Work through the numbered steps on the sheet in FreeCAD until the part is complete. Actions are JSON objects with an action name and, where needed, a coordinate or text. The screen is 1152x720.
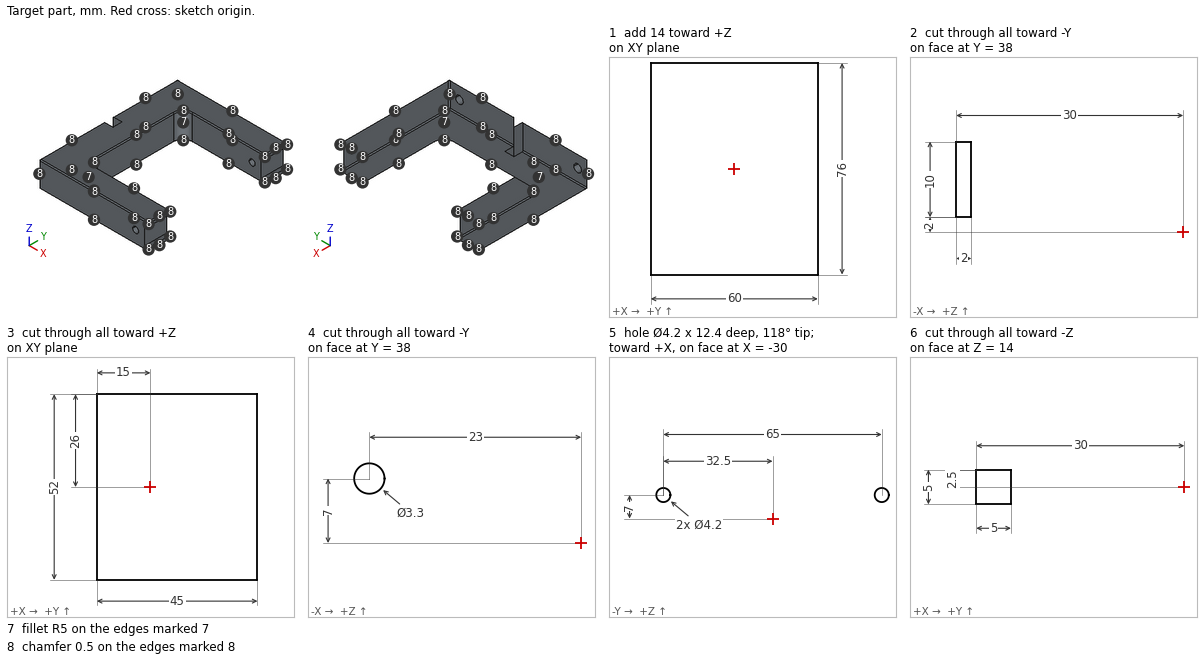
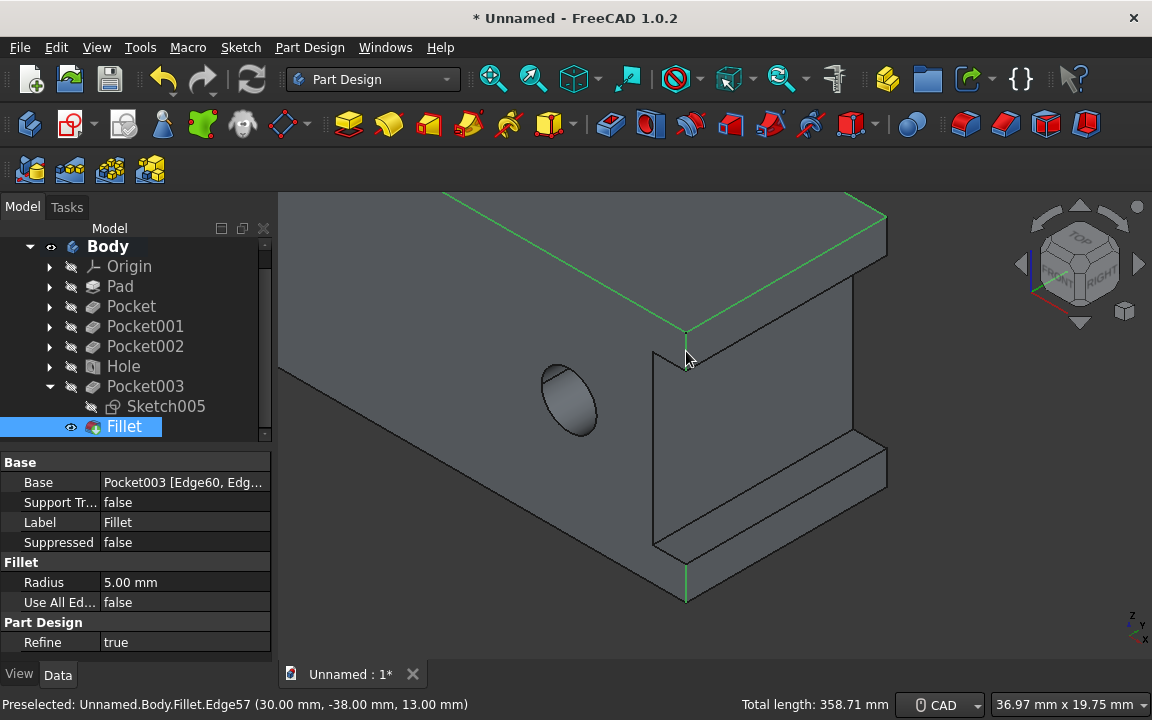
{"action": "key", "text": "v f"}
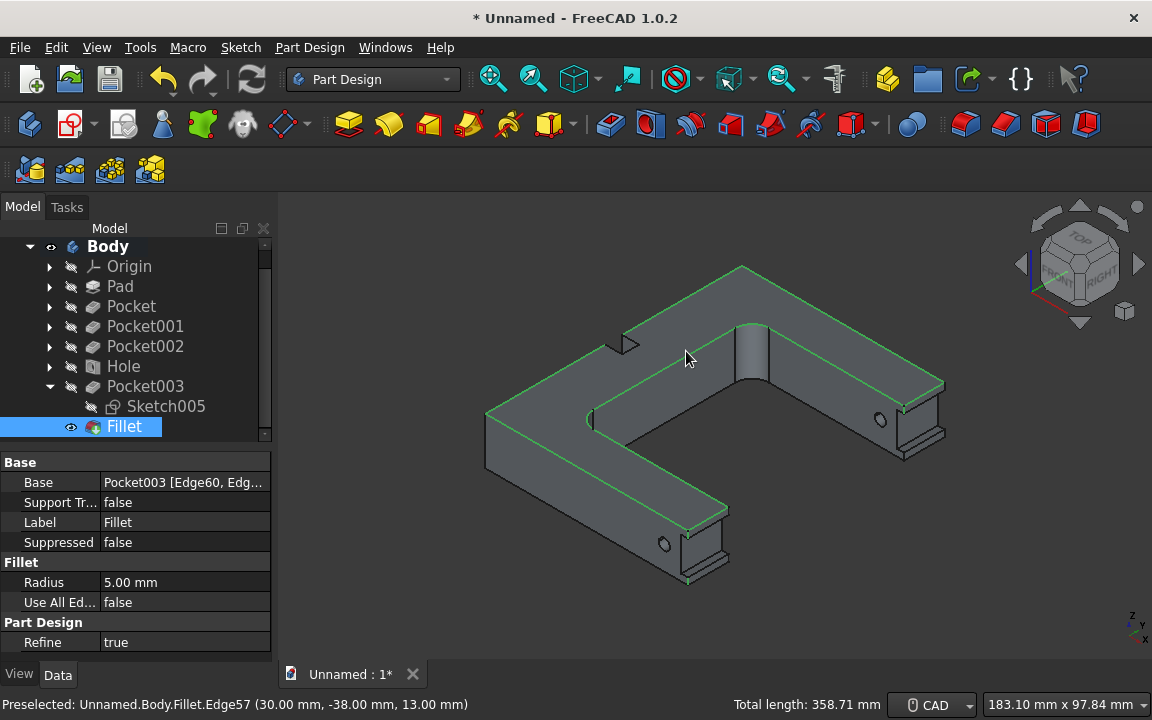
{"action": "key", "text": "1"}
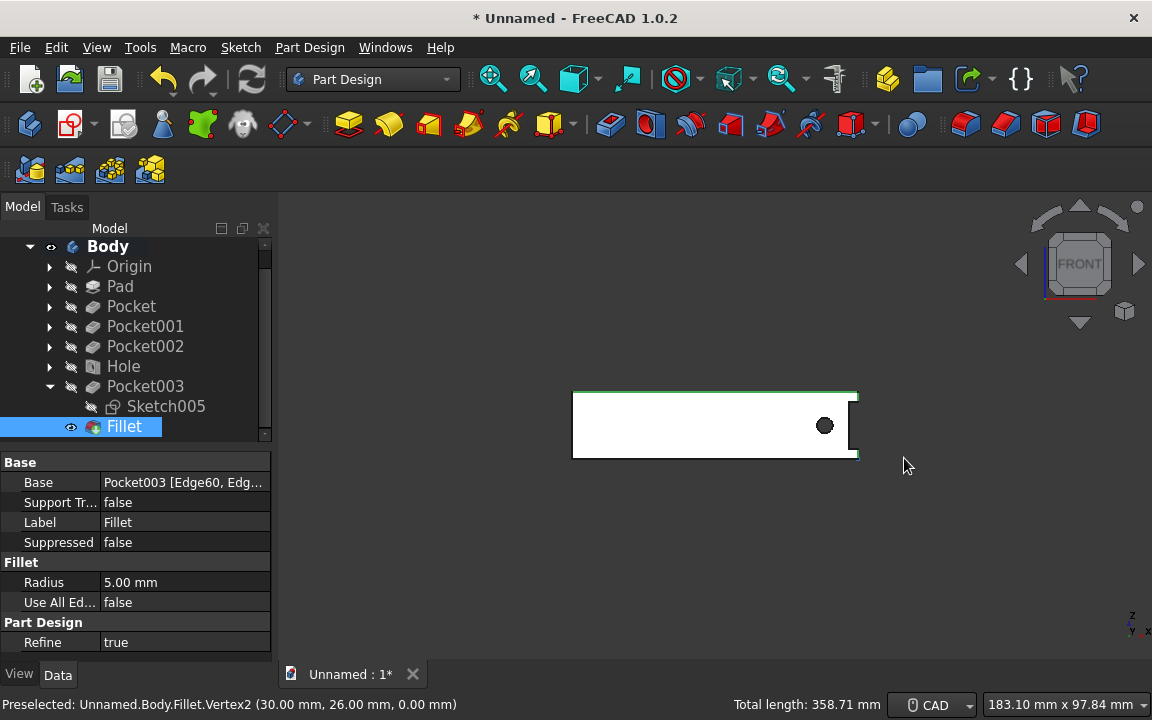
{"action": "key", "text": "v f"}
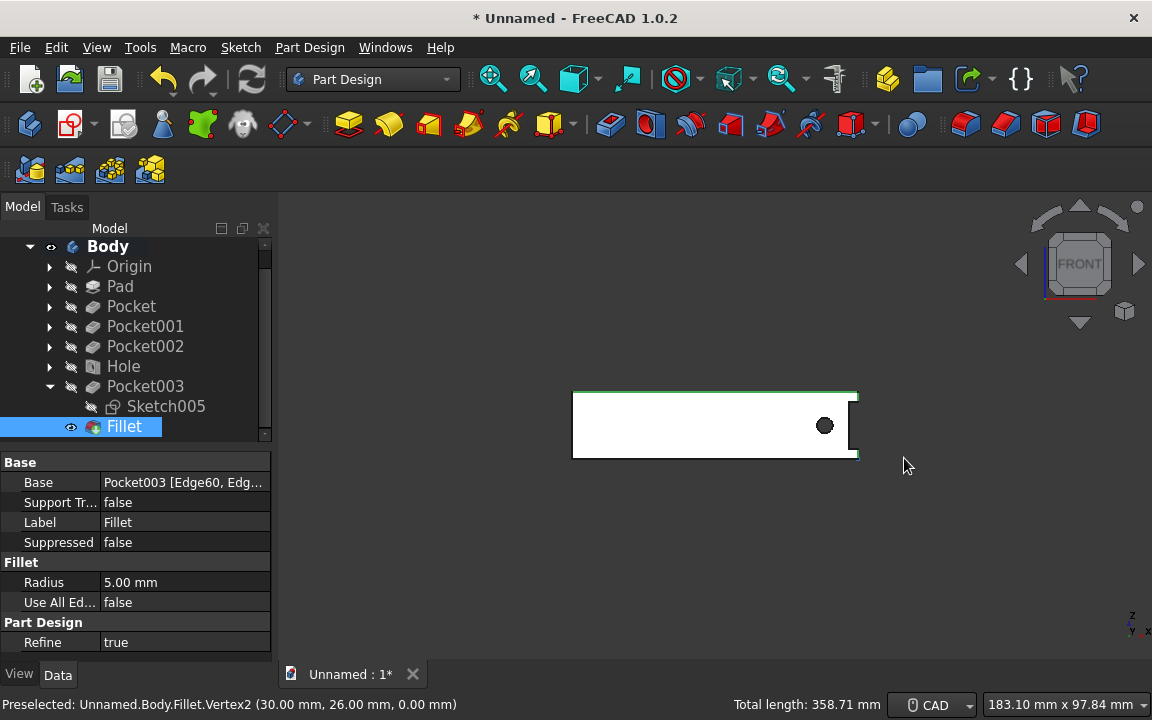
{"action": "left_click", "coordinate": [715, 458], "text": "ctrl"}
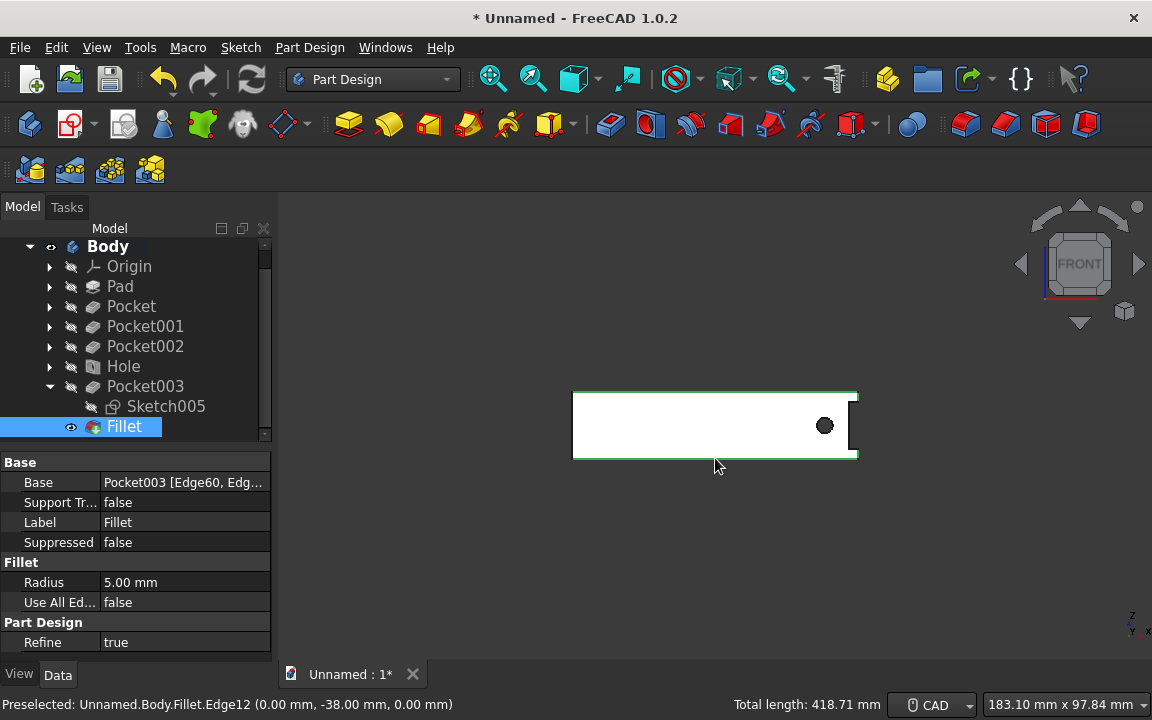
{"action": "left_click", "coordinate": [572, 425], "text": "ctrl"}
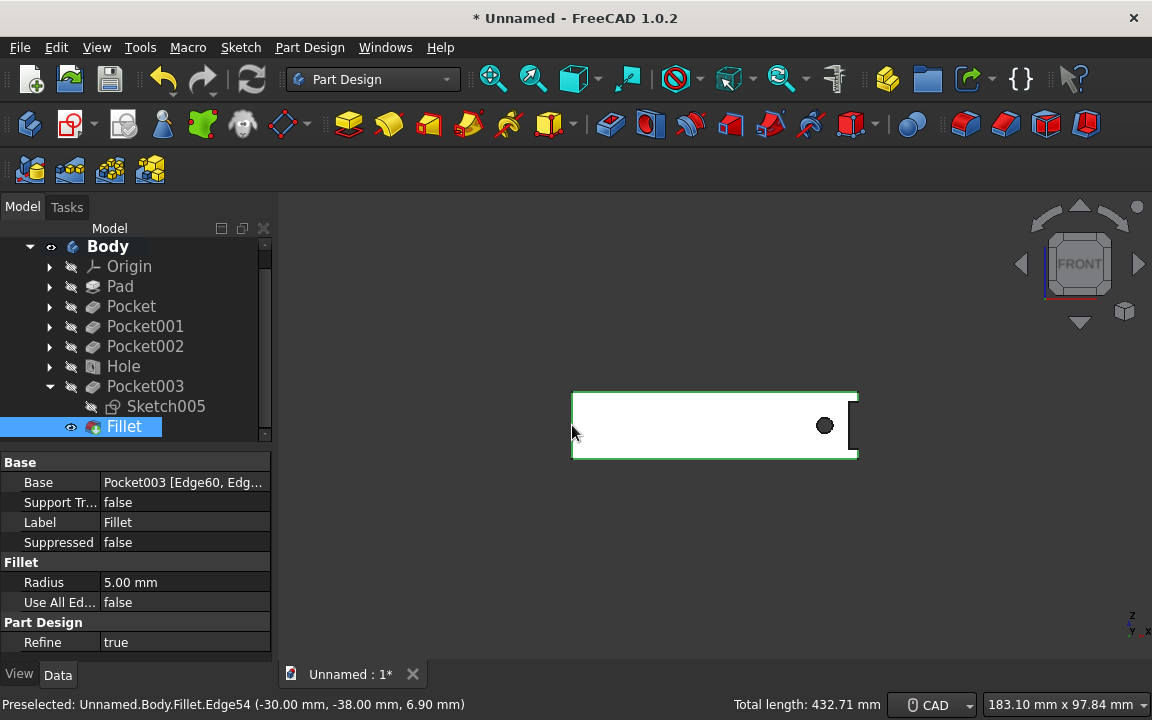
{"action": "scroll", "coordinate": [858, 453], "scroll_direction": "up", "scroll_amount": 8}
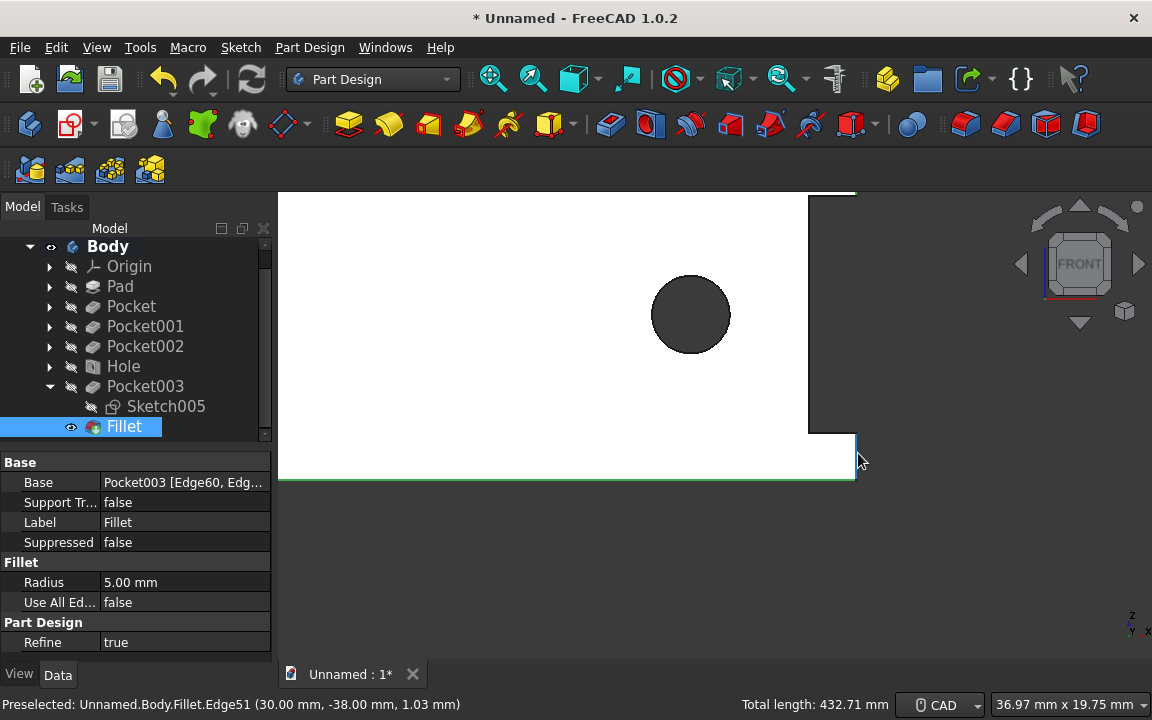
{"action": "key", "text": "v f"}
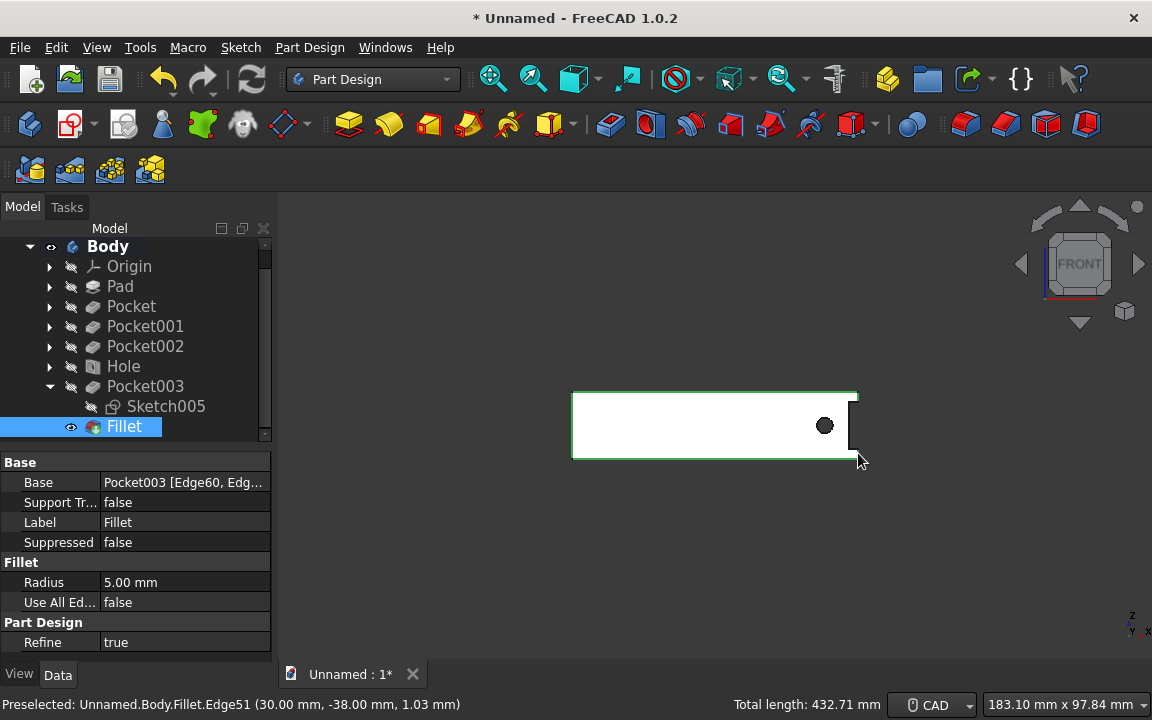
{"action": "key", "text": "3"}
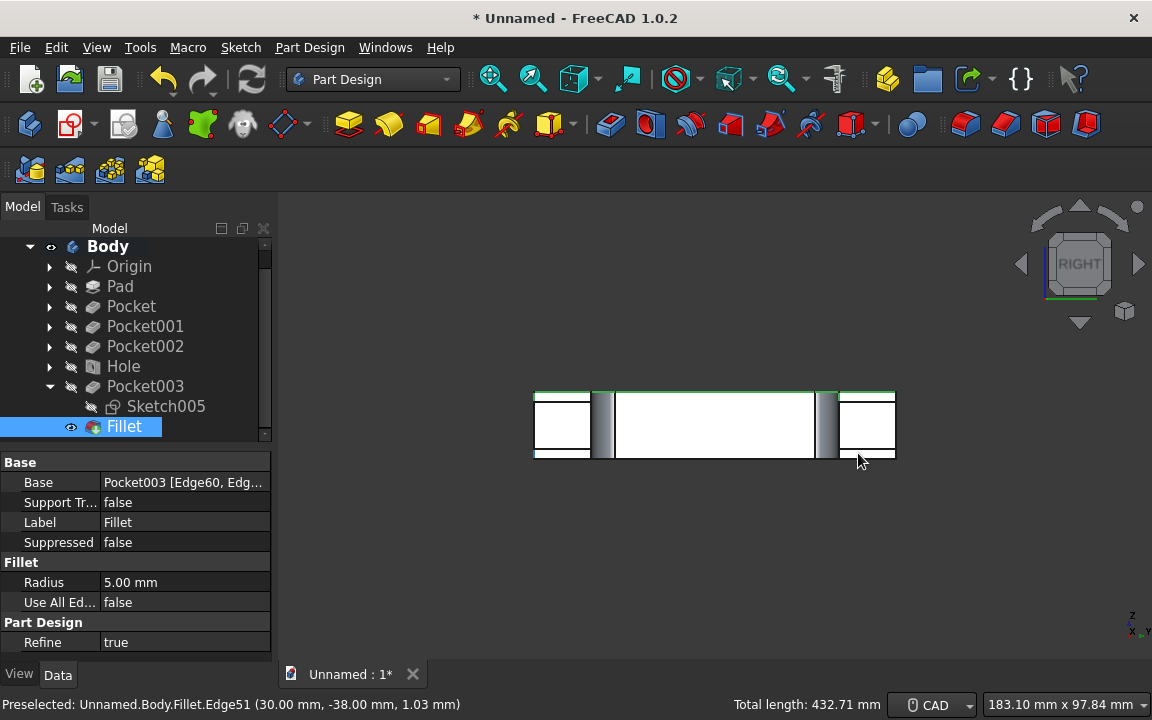
{"action": "key", "text": "v f"}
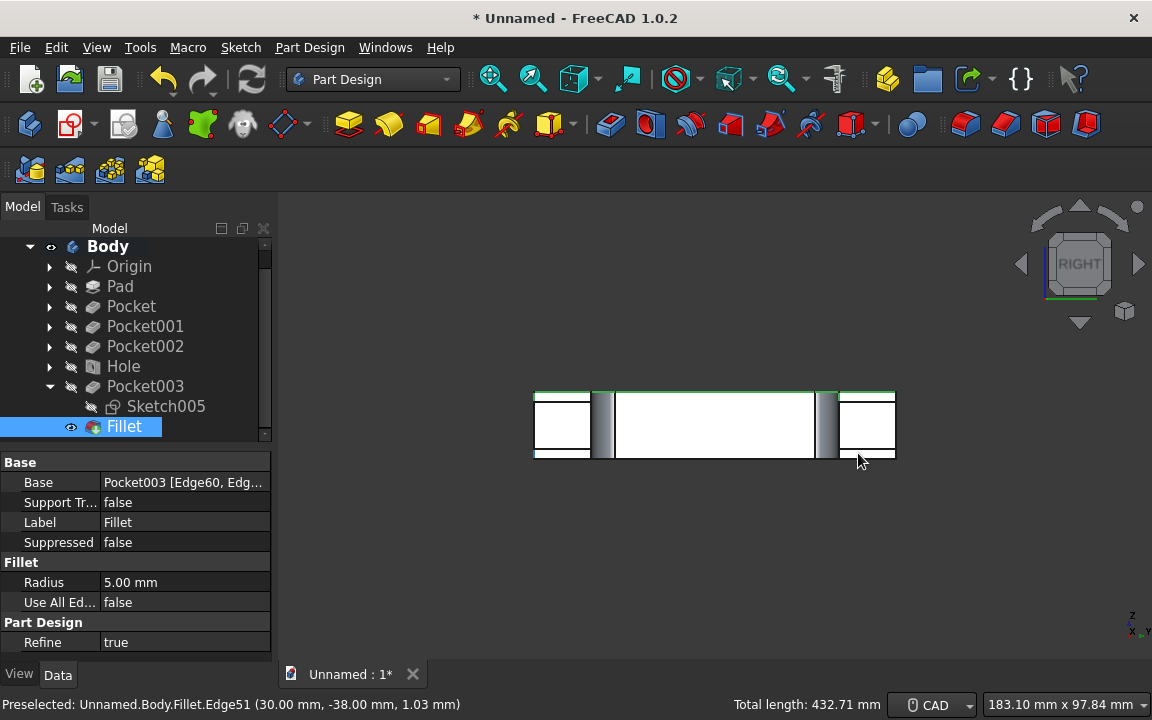
{"action": "left_click", "coordinate": [868, 458], "text": "ctrl"}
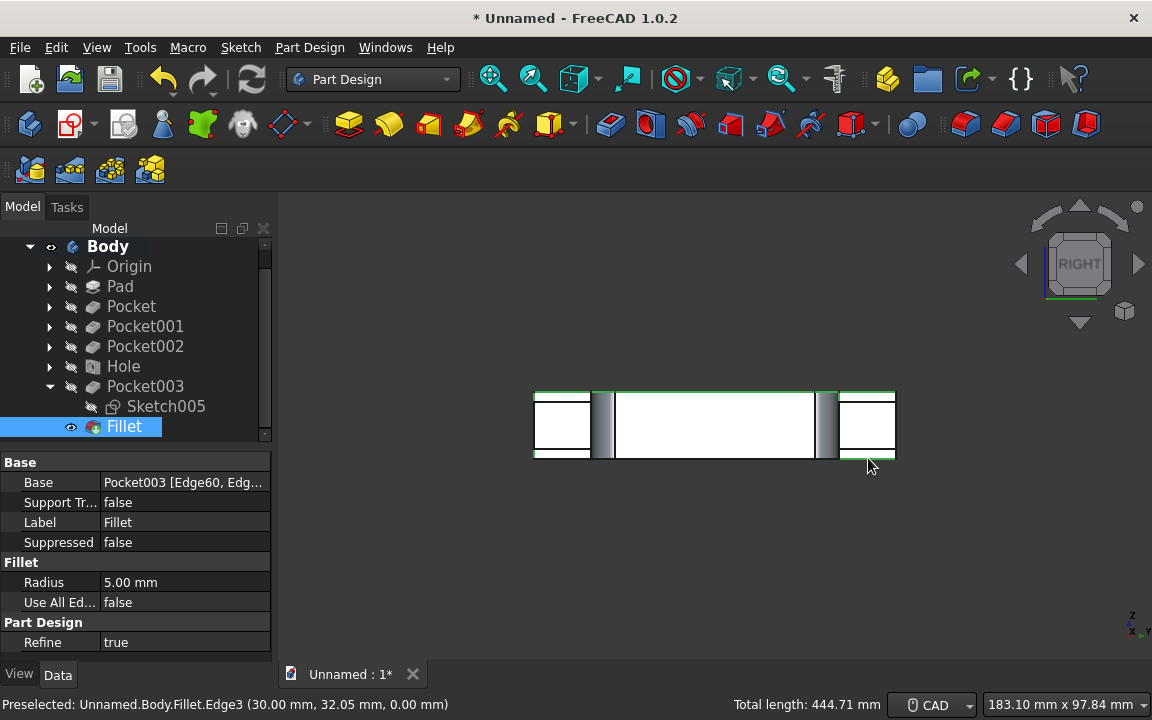
{"action": "left_click", "coordinate": [562, 458], "text": "ctrl"}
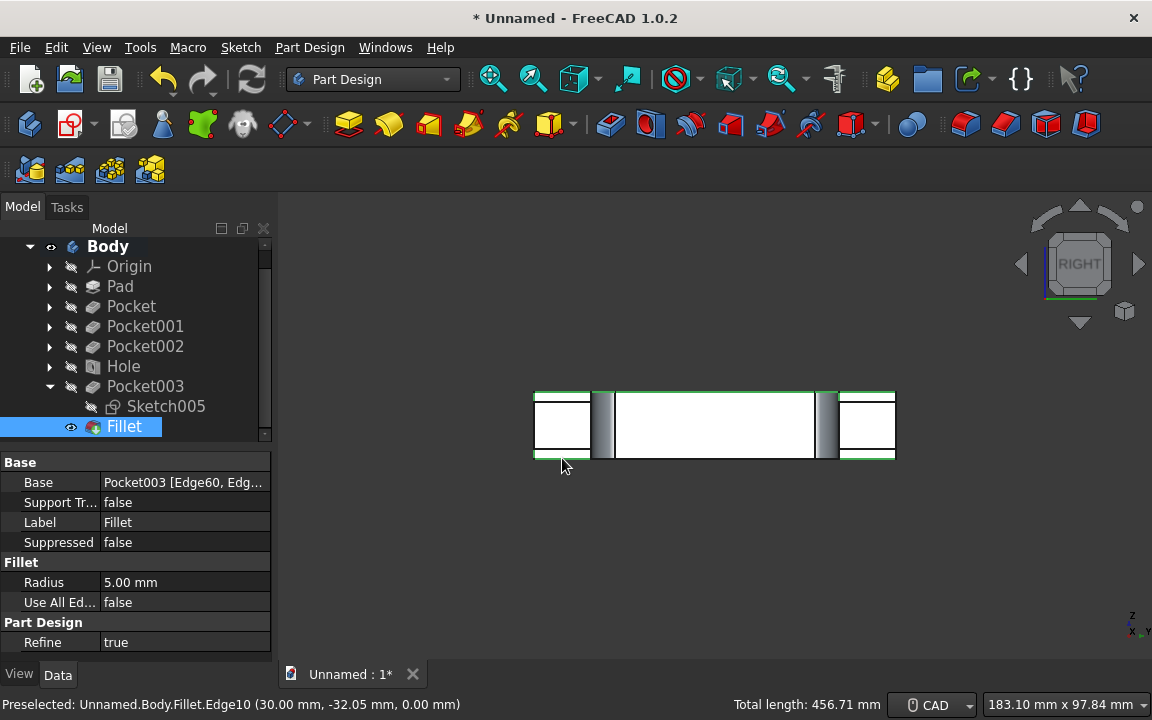
{"action": "left_click", "coordinate": [715, 458], "text": "ctrl"}